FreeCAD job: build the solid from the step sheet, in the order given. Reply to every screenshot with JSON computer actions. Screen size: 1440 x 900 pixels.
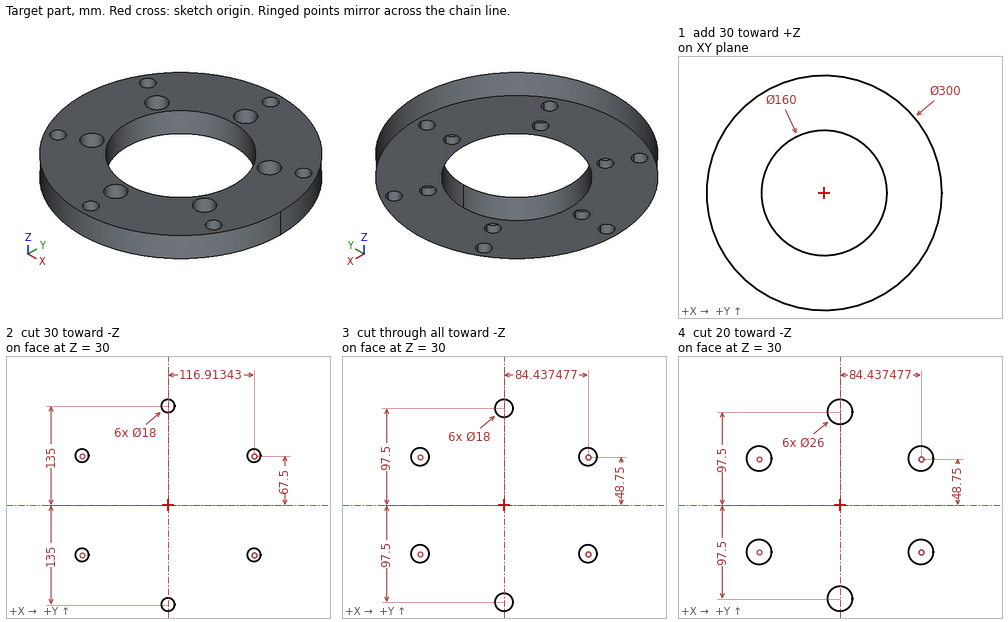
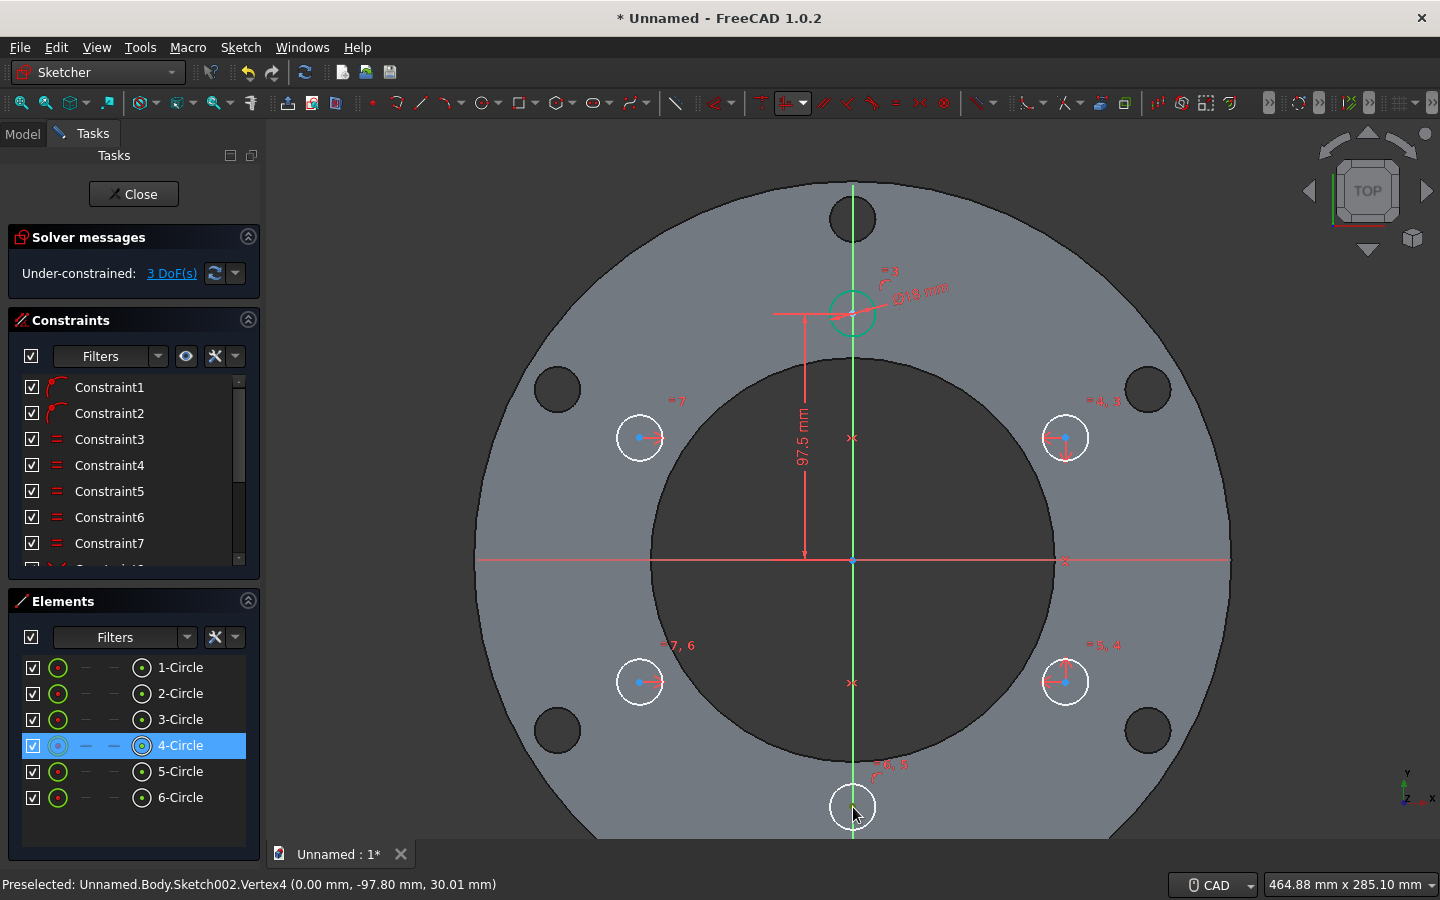
{"action": "left_click", "coordinate": [734, 104]}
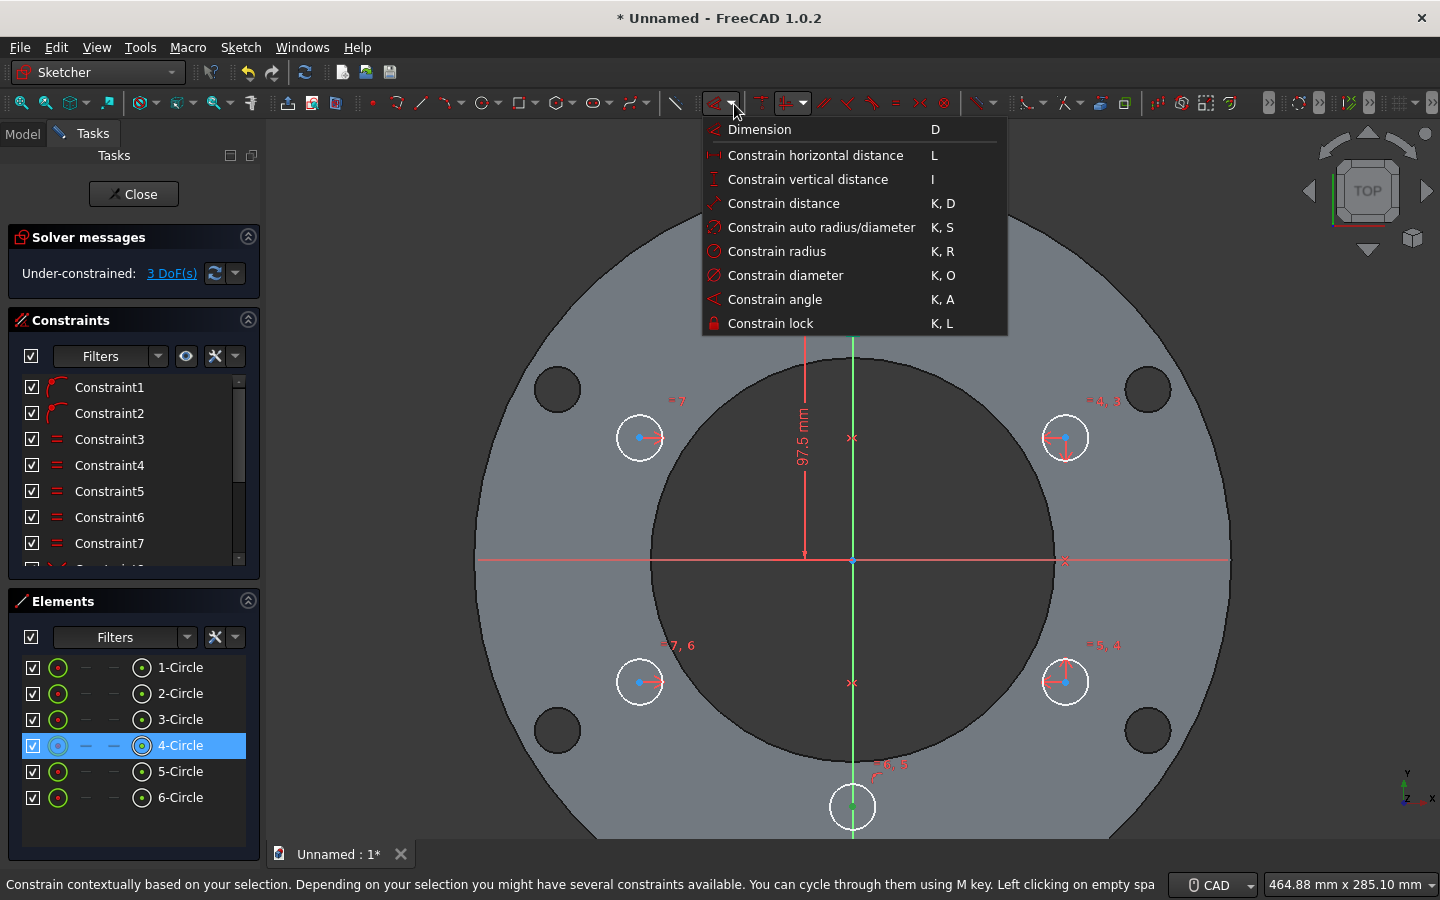
{"action": "left_click", "coordinate": [855, 179]}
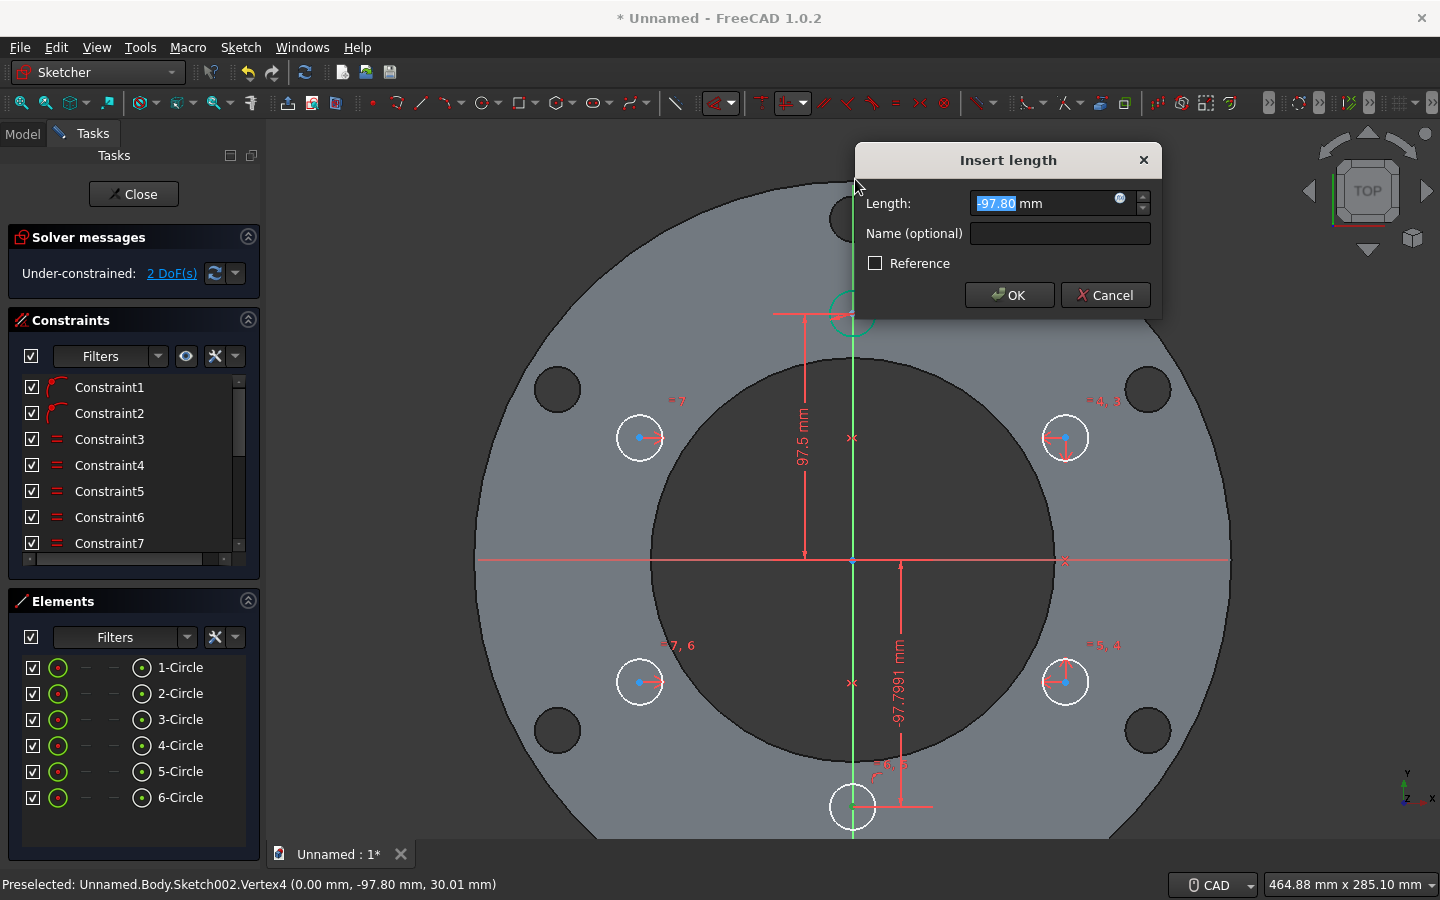
{"action": "type", "text": "-97.5"}
{"action": "key", "text": "Return"}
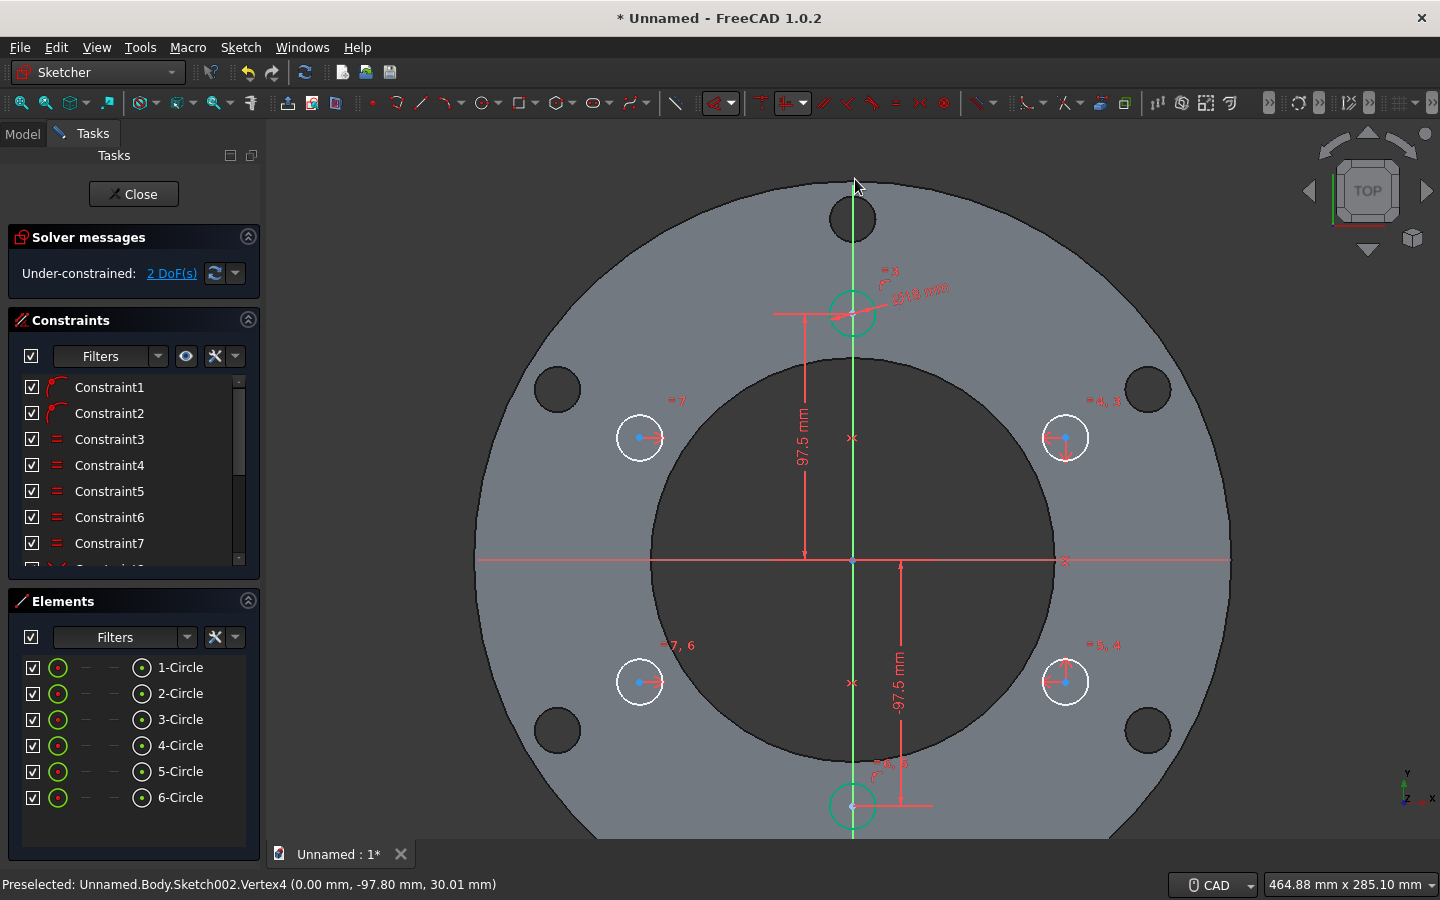
{"action": "left_click", "coordinate": [1066, 438]}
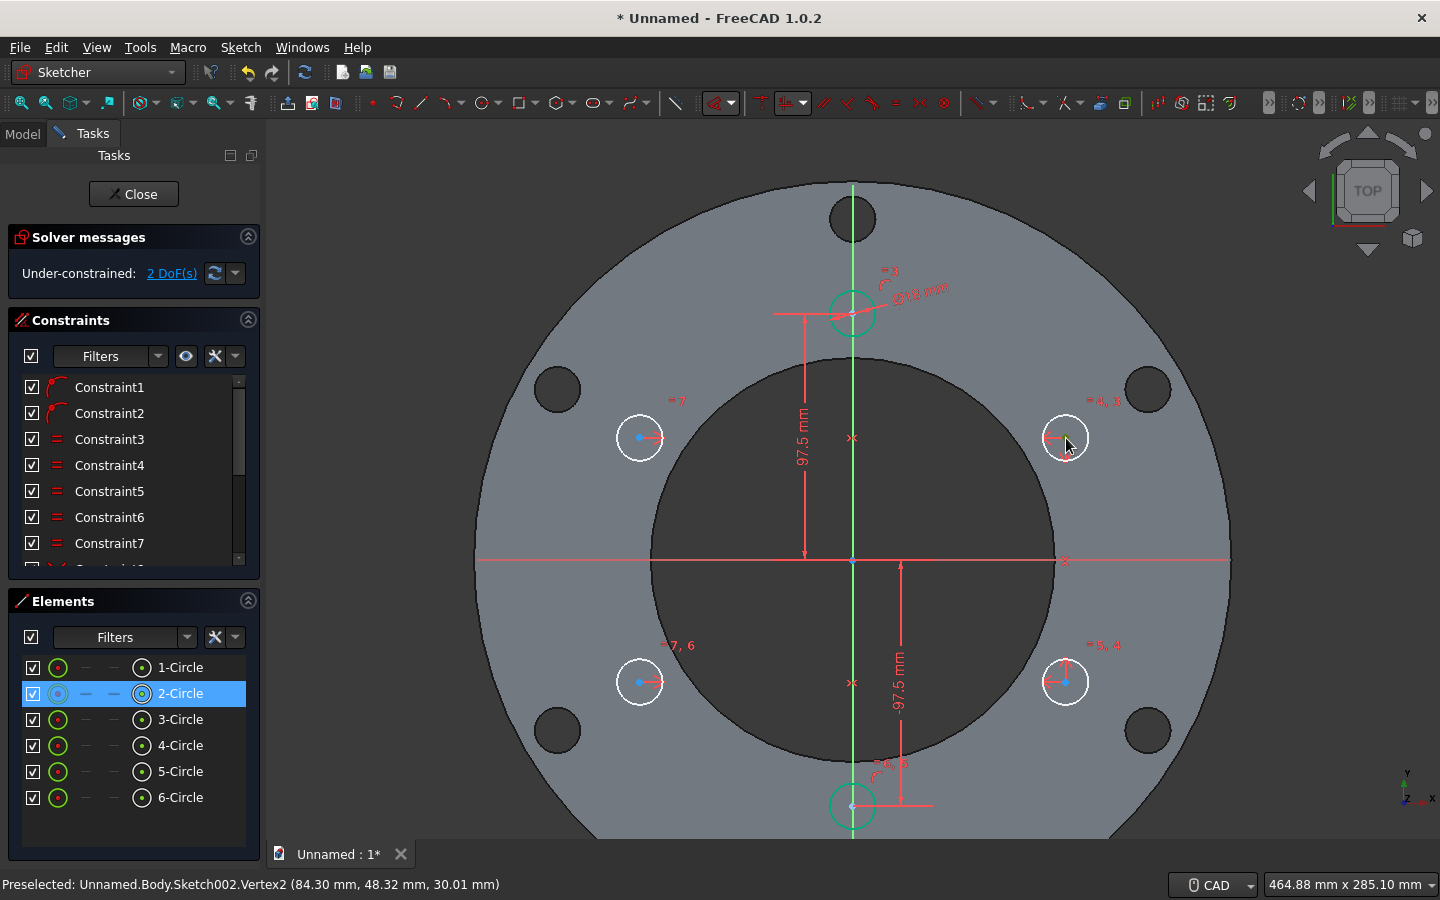
{"action": "key", "text": "i"}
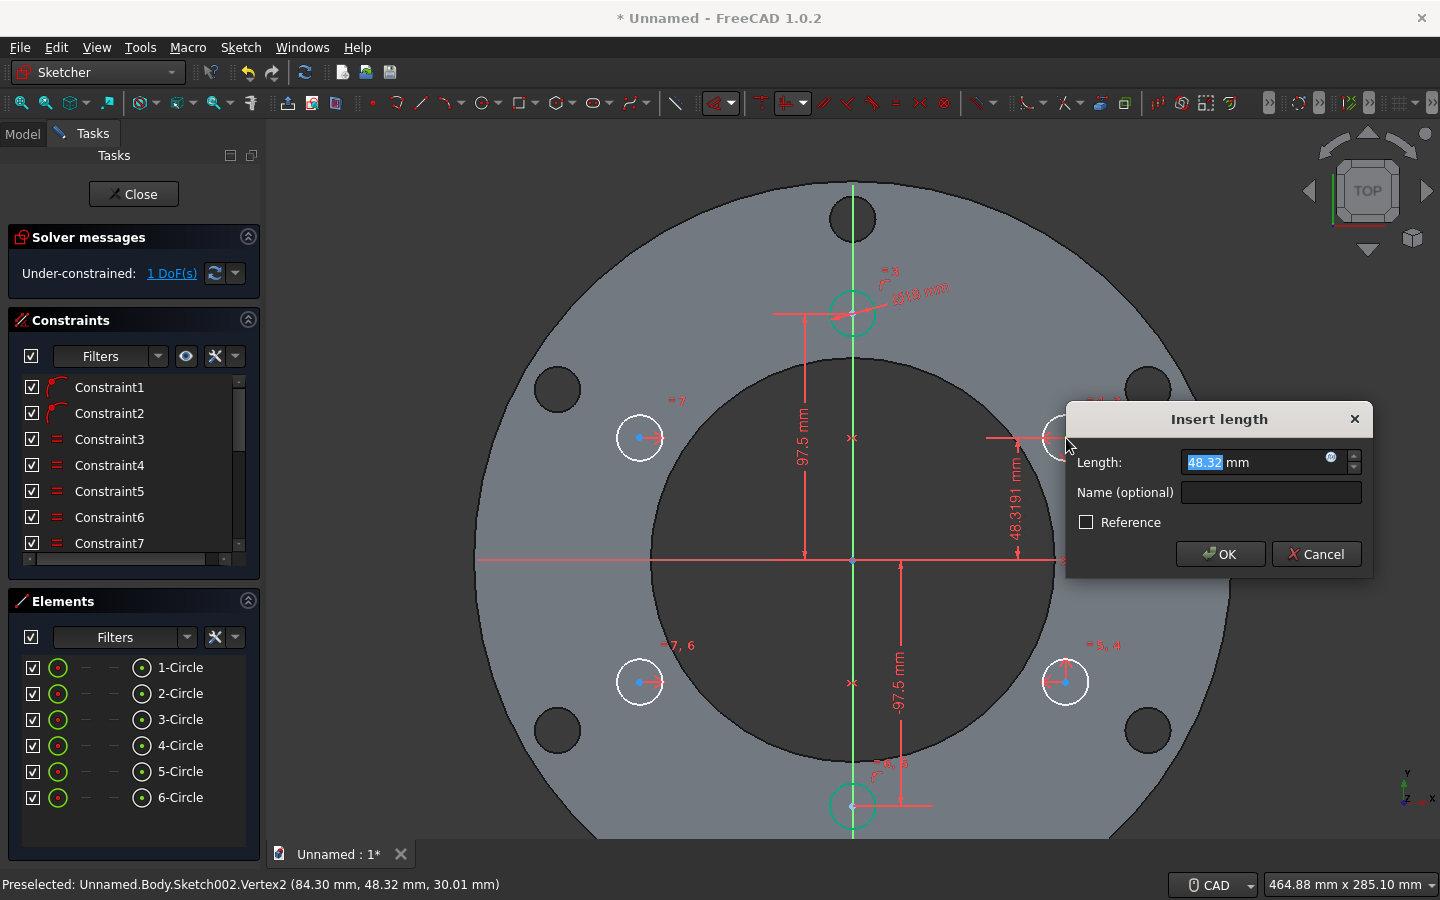
{"action": "type", "text": "48.75"}
{"action": "key", "text": "Return"}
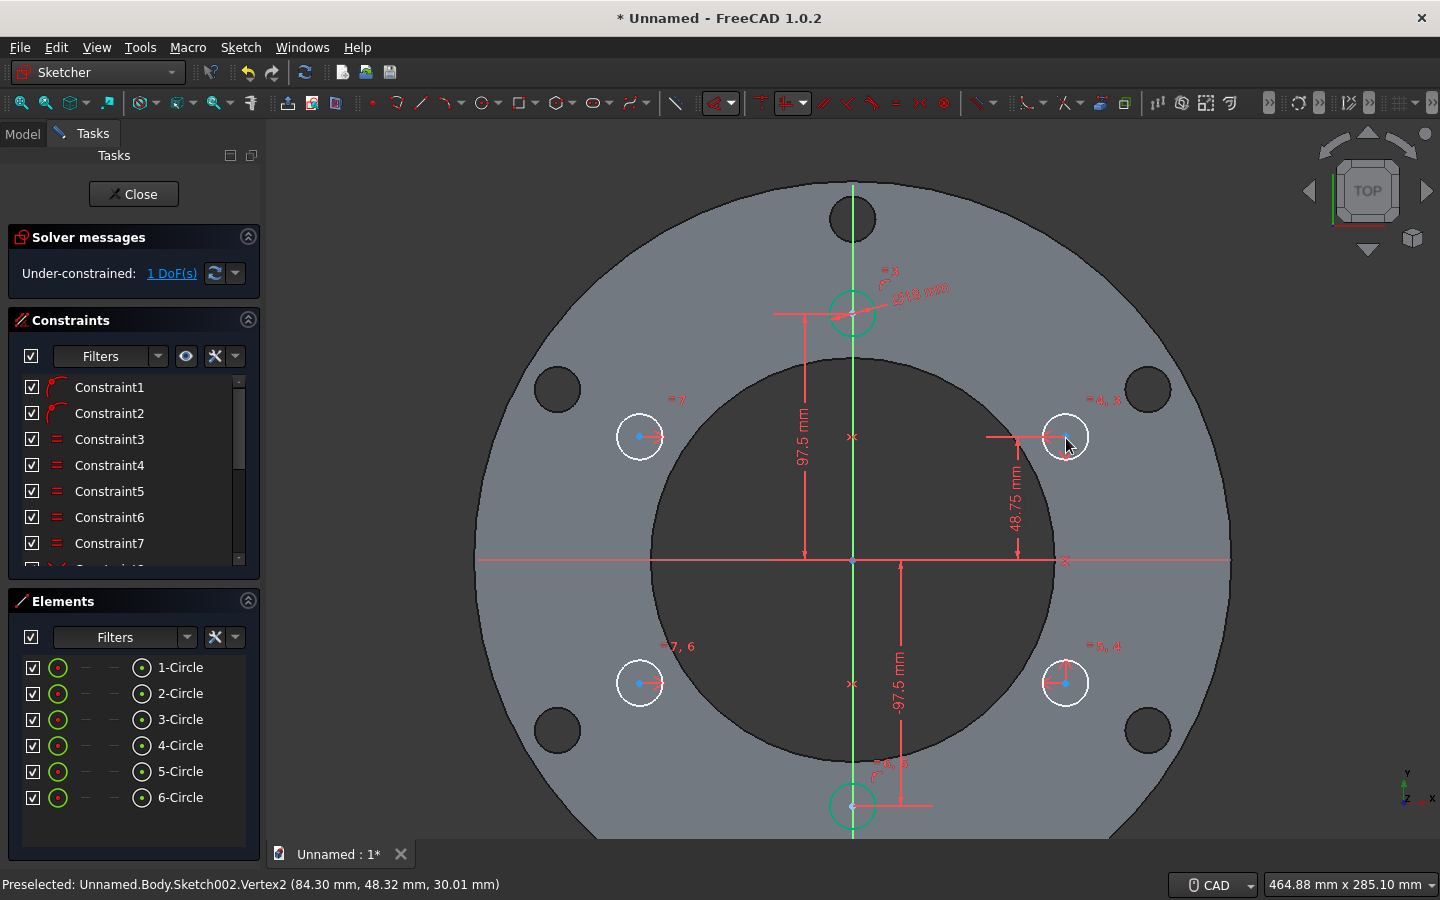
{"action": "left_click", "coordinate": [1066, 437]}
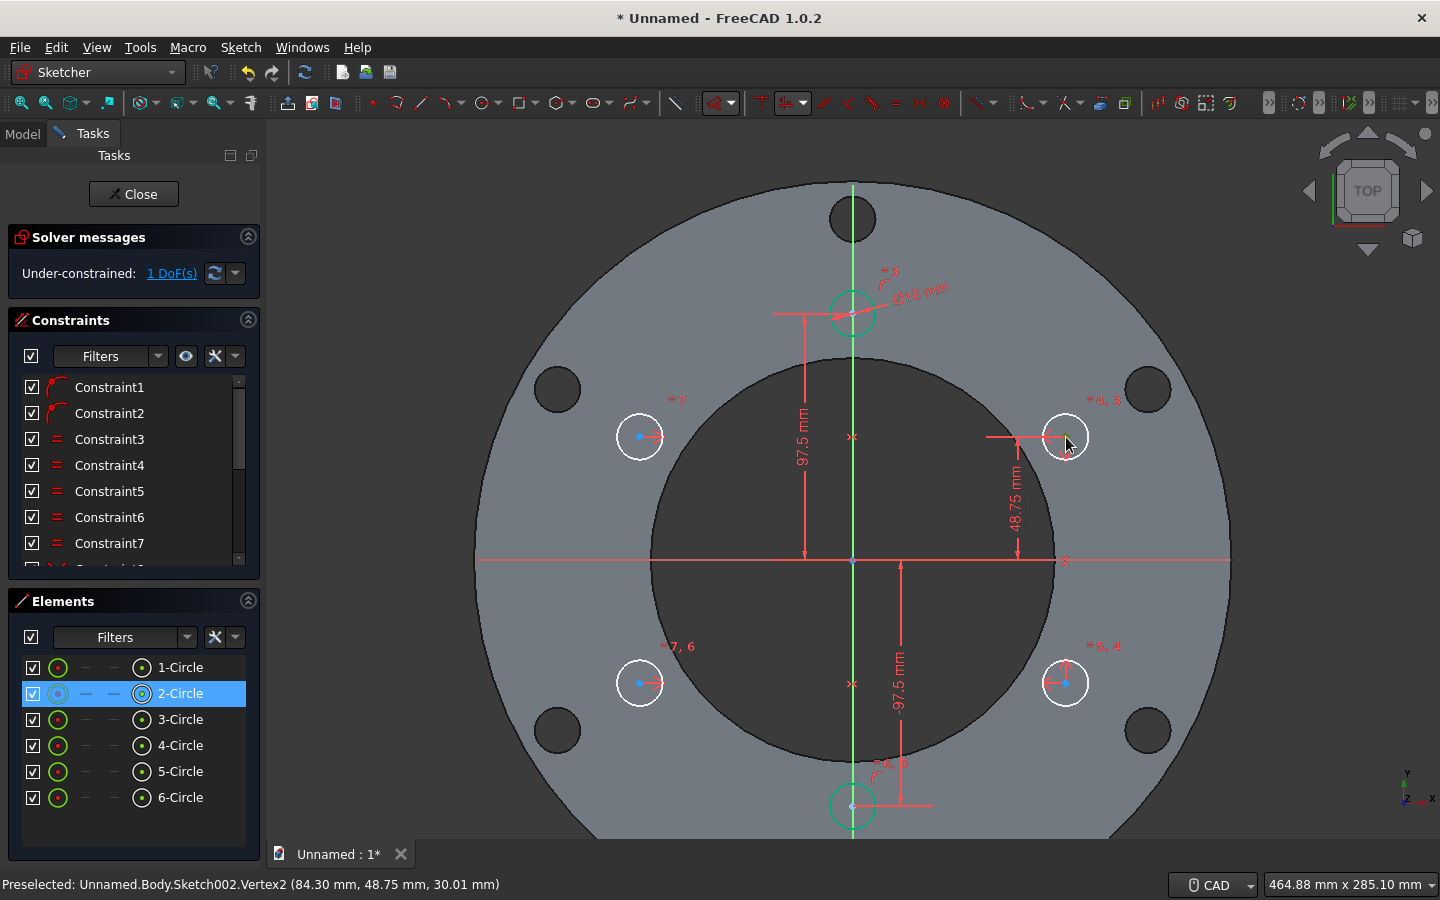
{"action": "left_click", "coordinate": [734, 104]}